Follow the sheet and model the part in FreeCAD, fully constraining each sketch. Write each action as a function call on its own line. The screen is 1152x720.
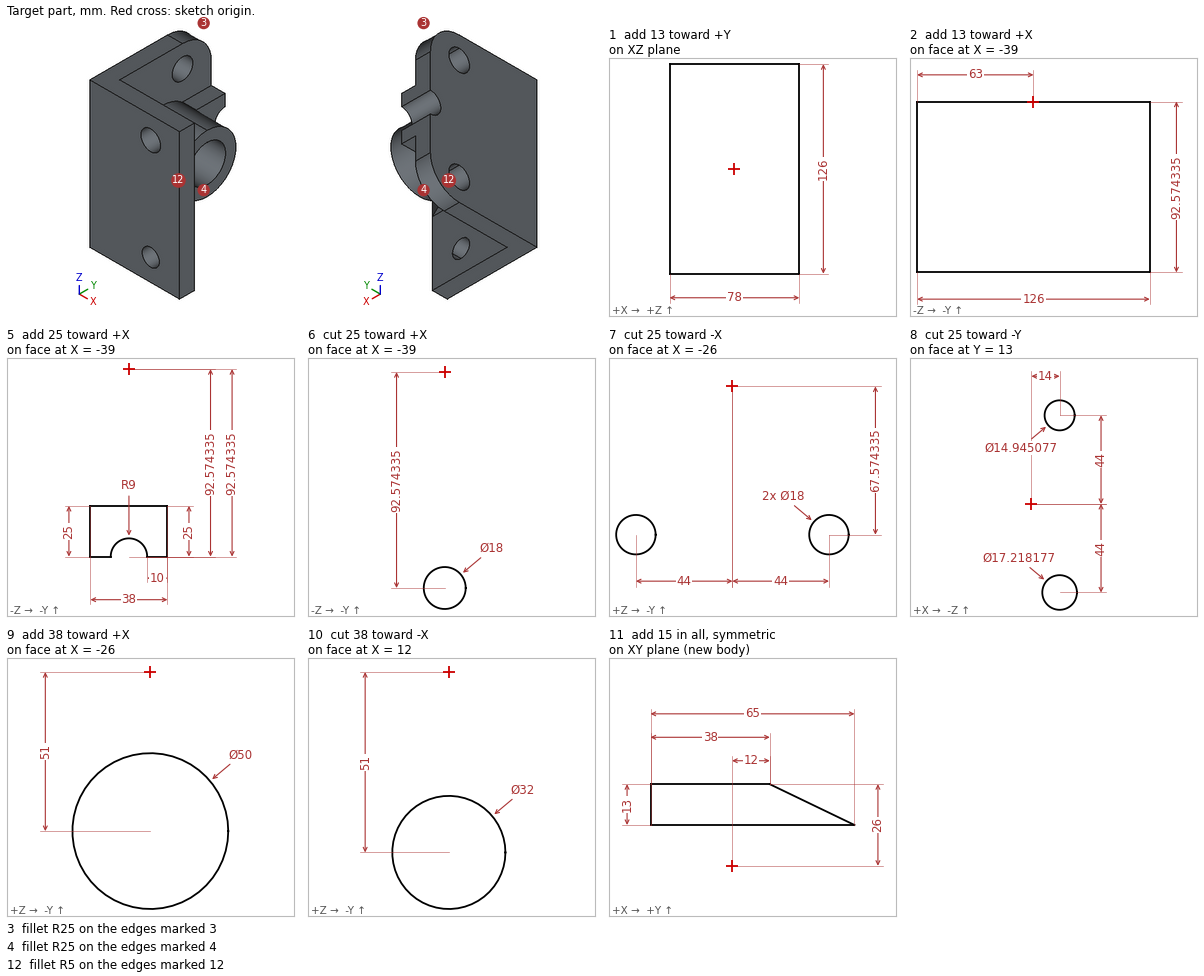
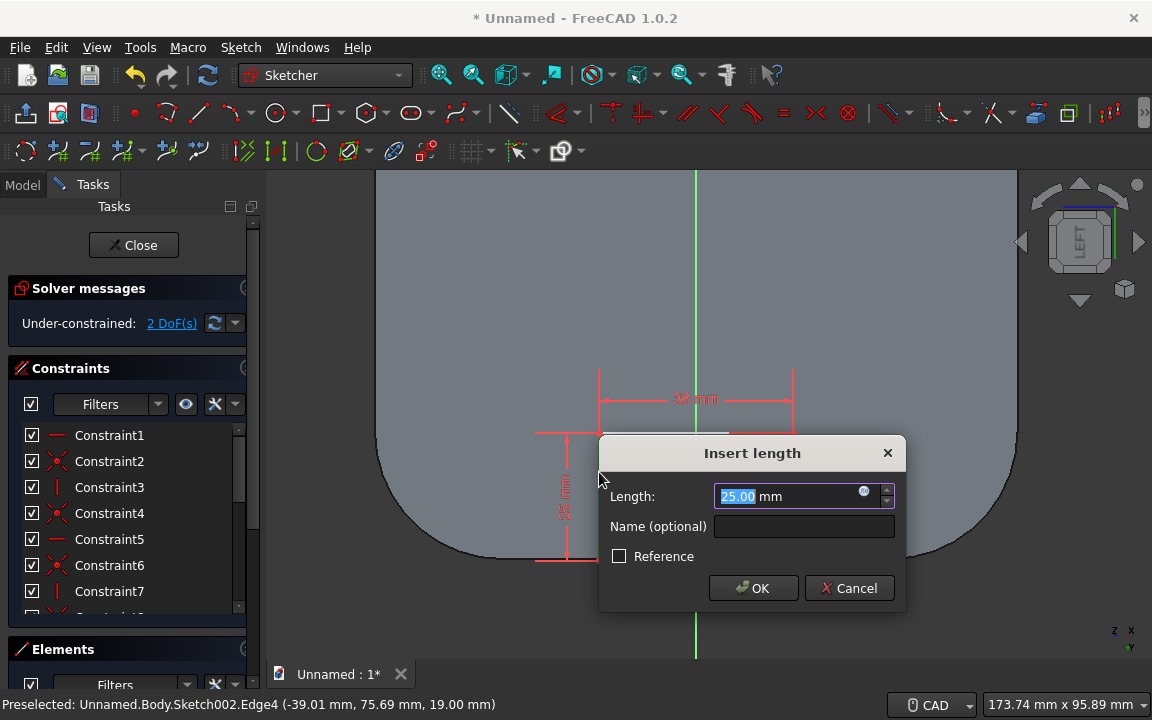
text(25)
key(Return)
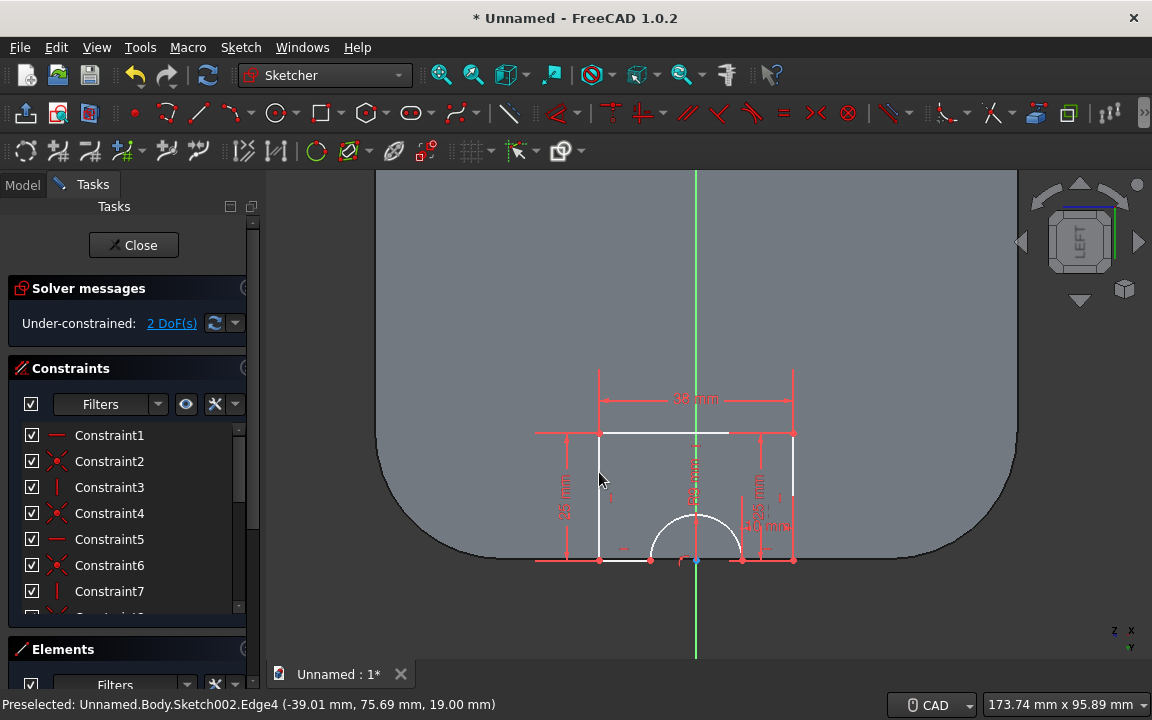
click(742, 561)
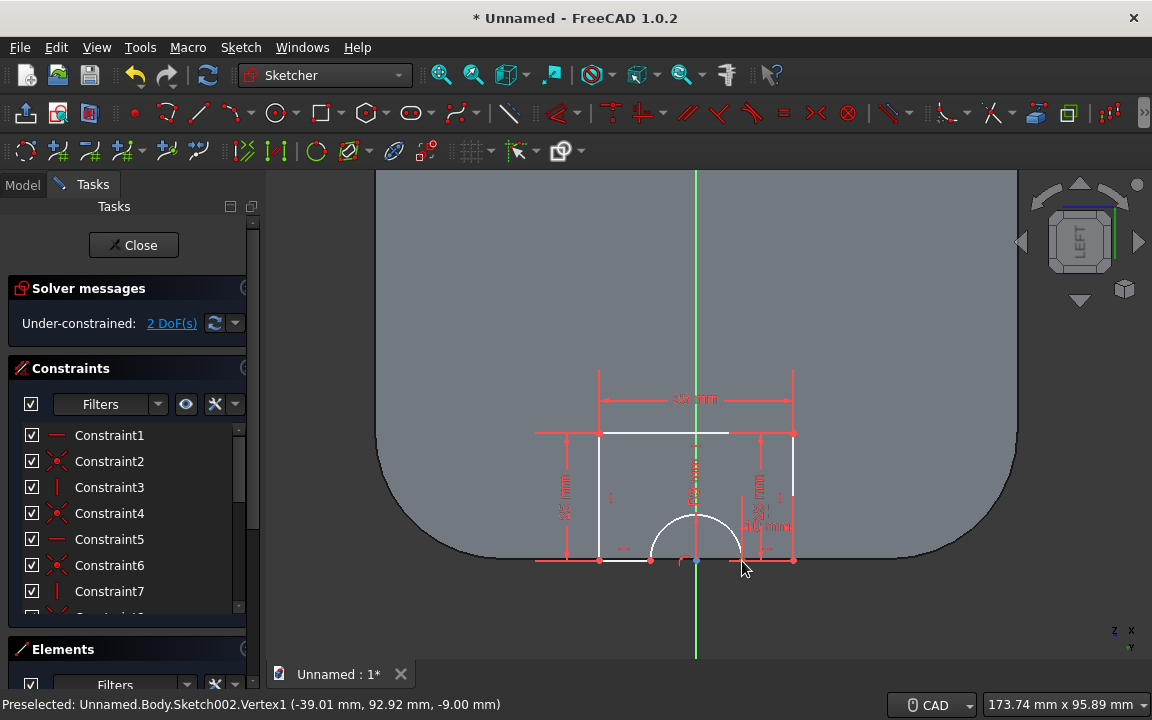
key(i)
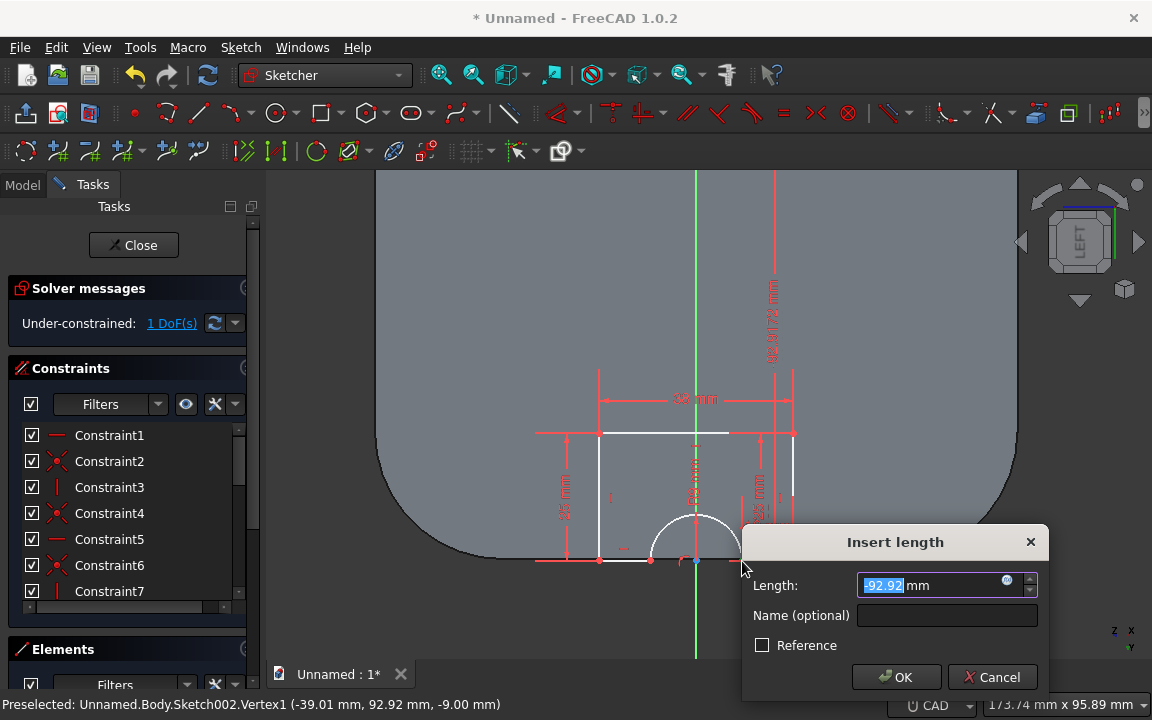
text(-92.574335)
key(Return)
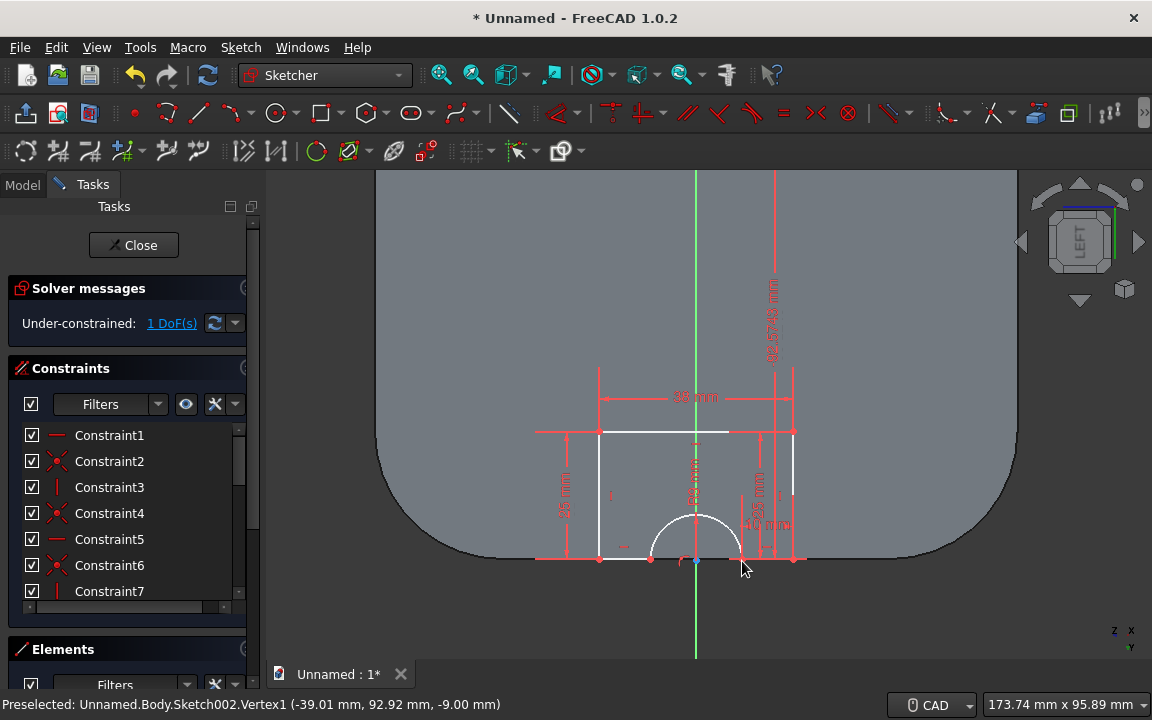
click(696, 561)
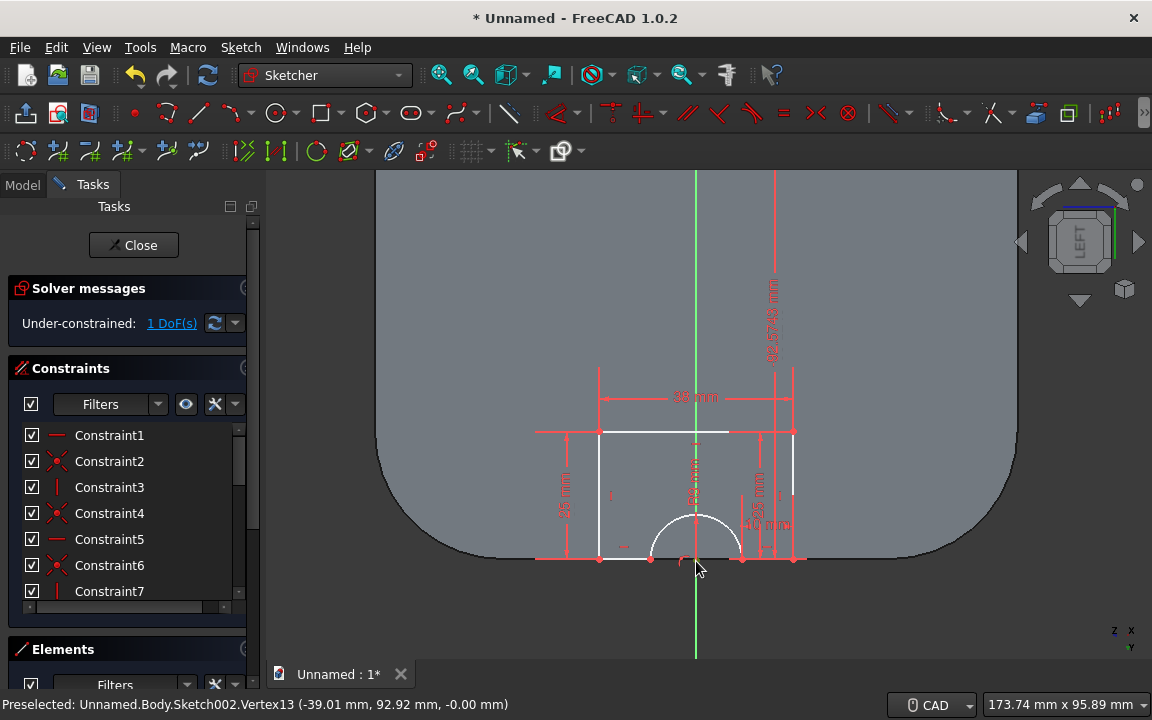
key(i)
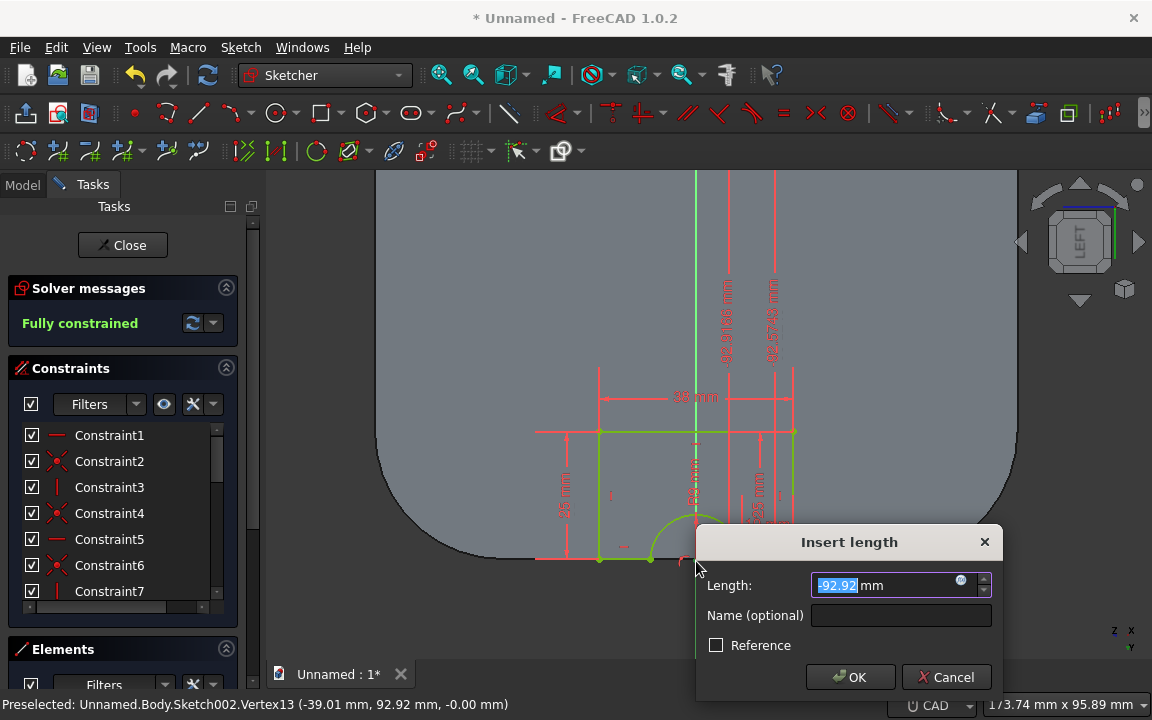
text(-92.574335)
key(Return)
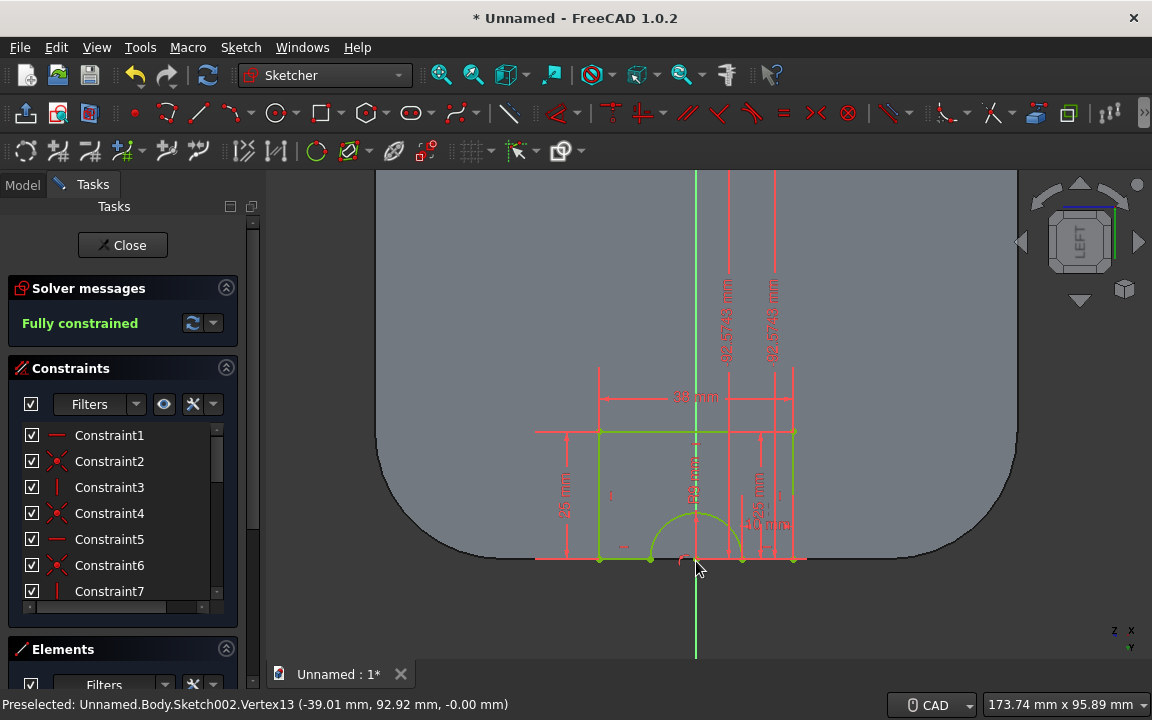
click(123, 245)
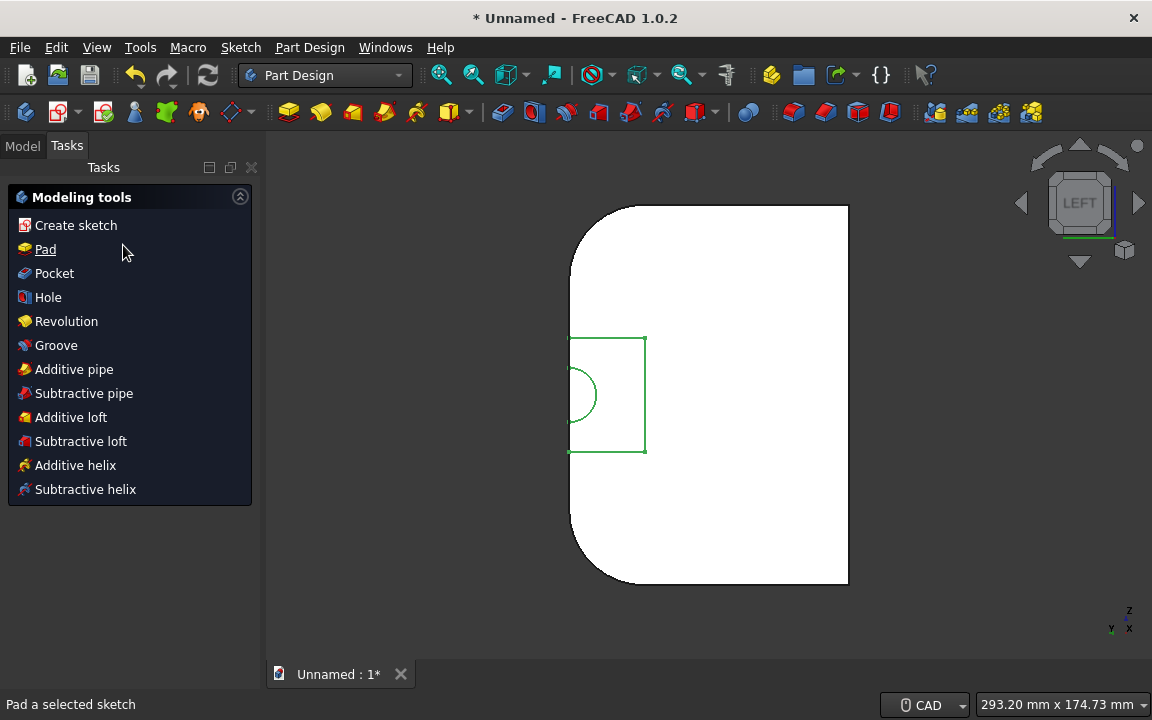
click(290, 112)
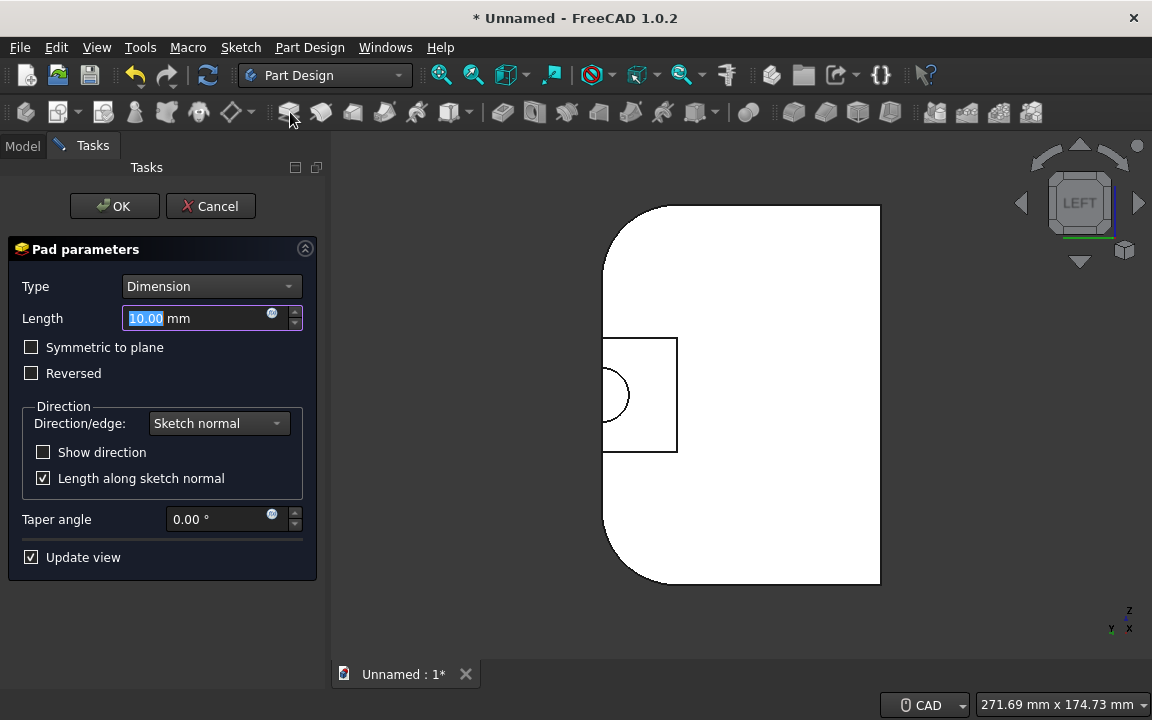
text(25)
key(Tab)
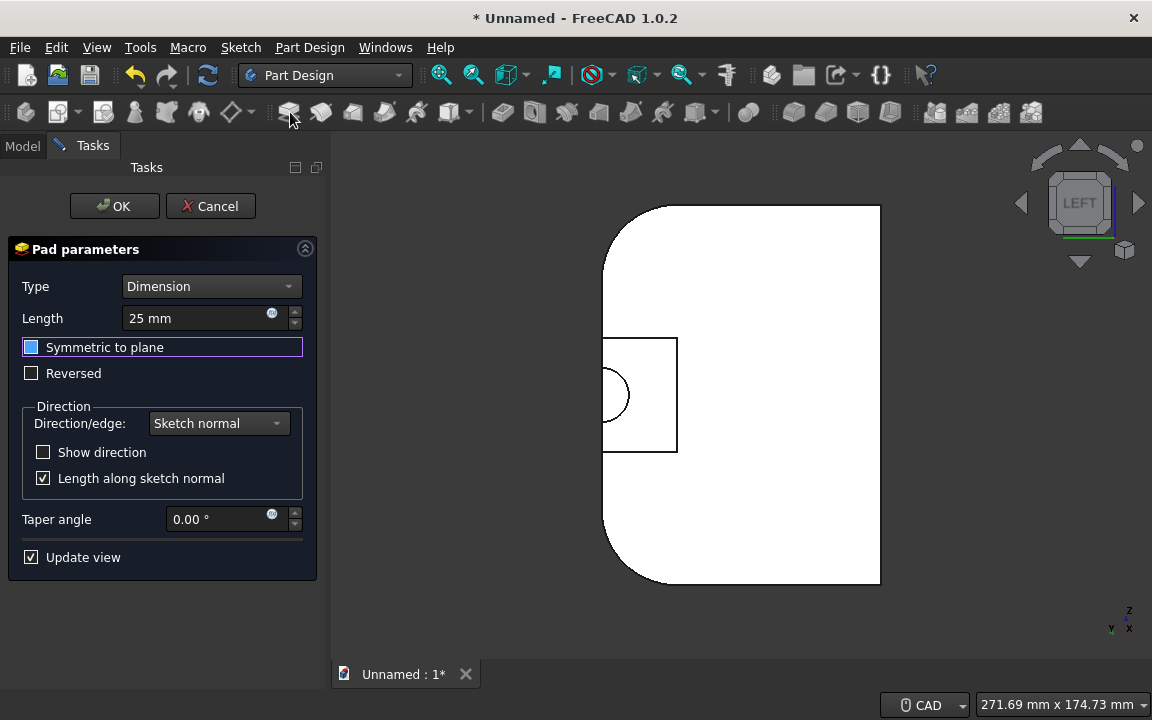
click(30, 373)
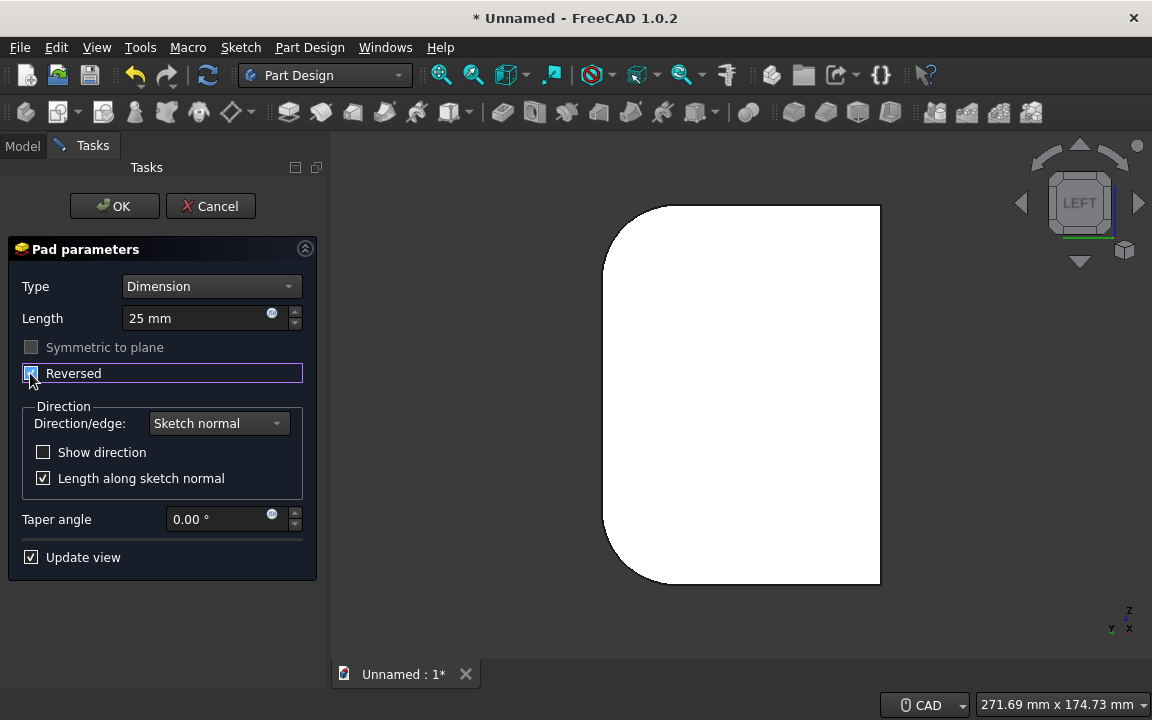
click(115, 206)